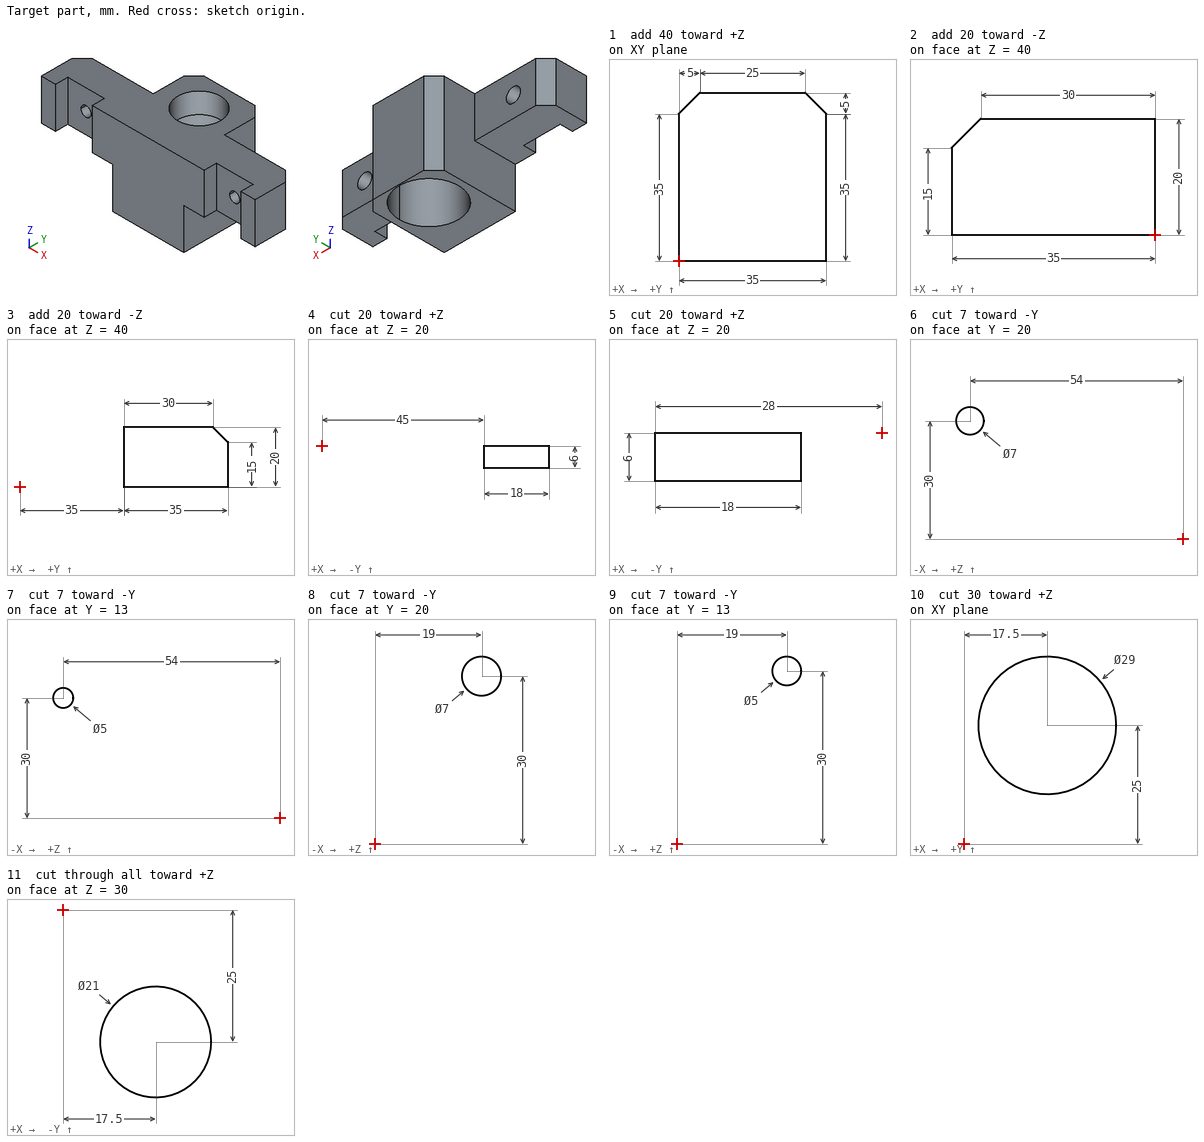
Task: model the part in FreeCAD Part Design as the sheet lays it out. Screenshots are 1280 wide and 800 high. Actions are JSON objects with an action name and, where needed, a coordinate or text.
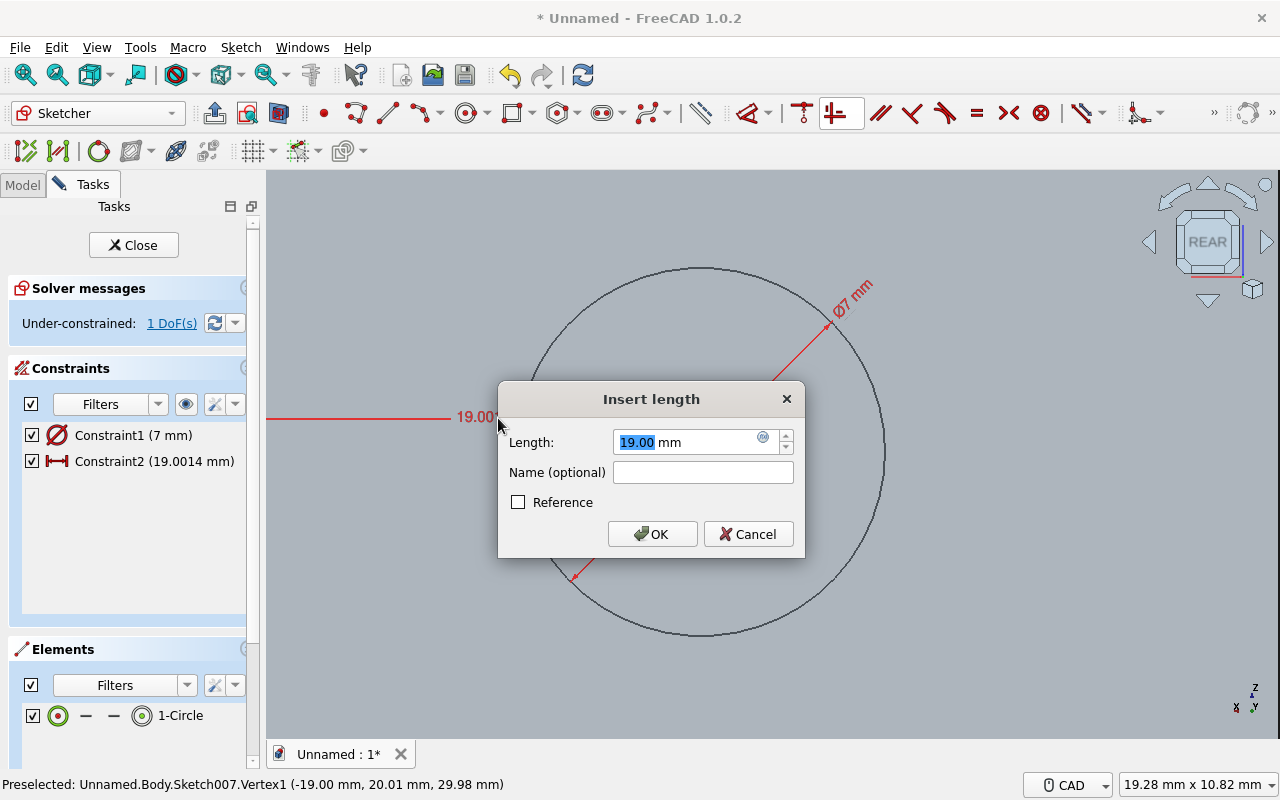
{"action": "type", "text": "19"}
{"action": "key", "text": "Return"}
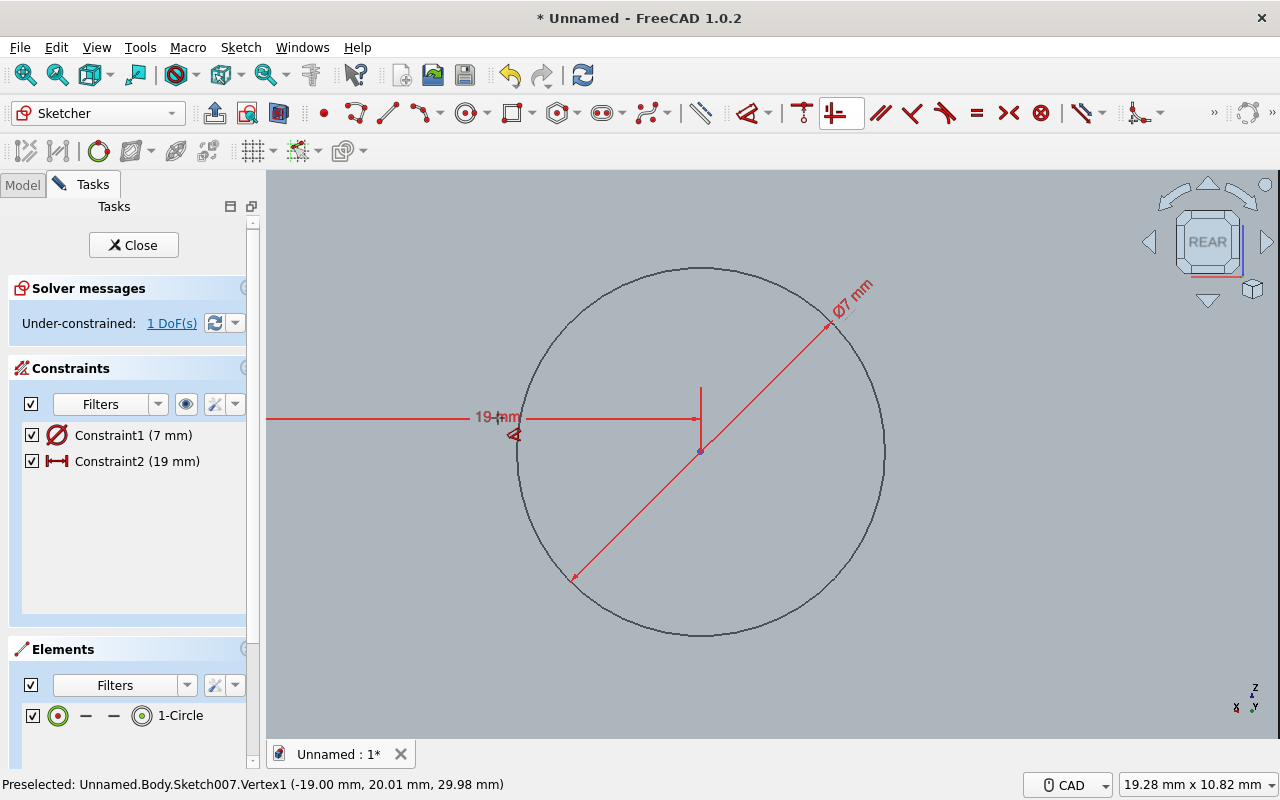
{"action": "left_click", "coordinate": [701, 452]}
{"action": "left_click", "coordinate": [735, 581]}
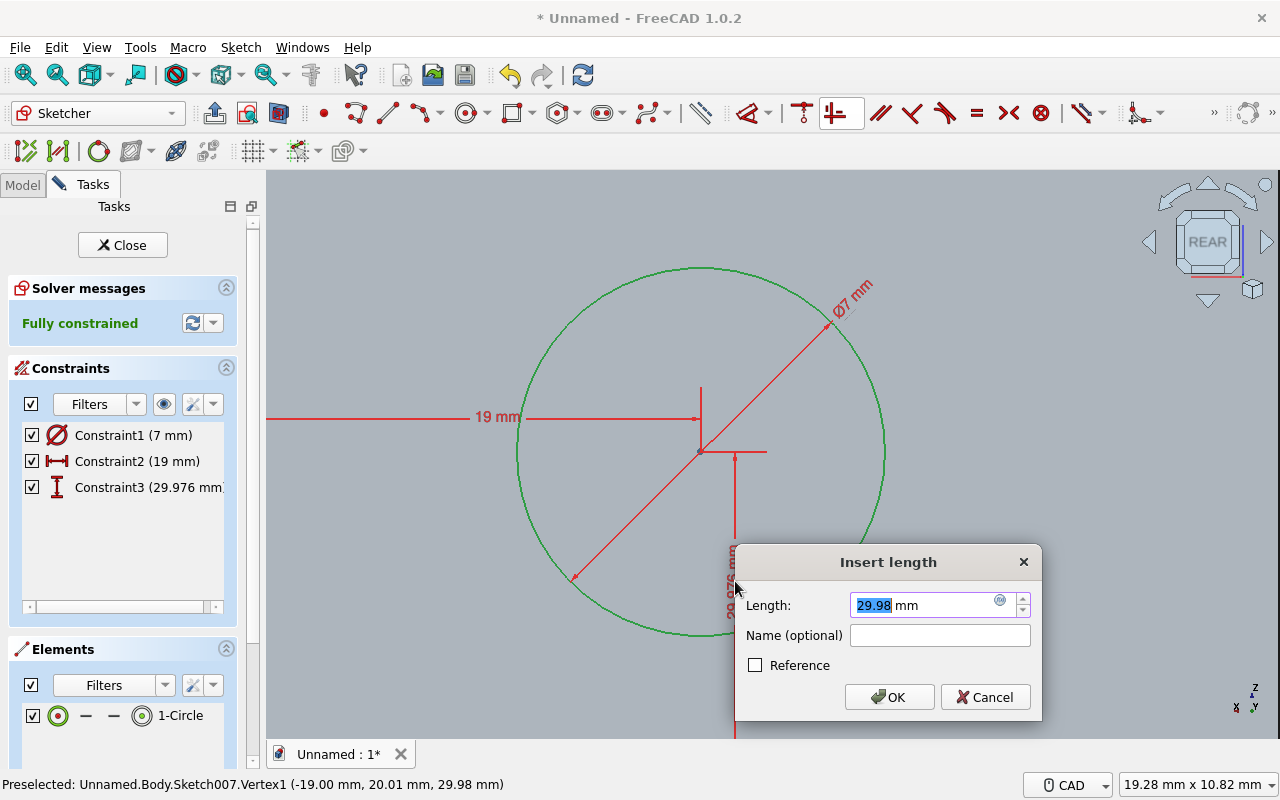
{"action": "type", "text": "30"}
{"action": "key", "text": "Return"}
{"action": "key", "text": "Escape"}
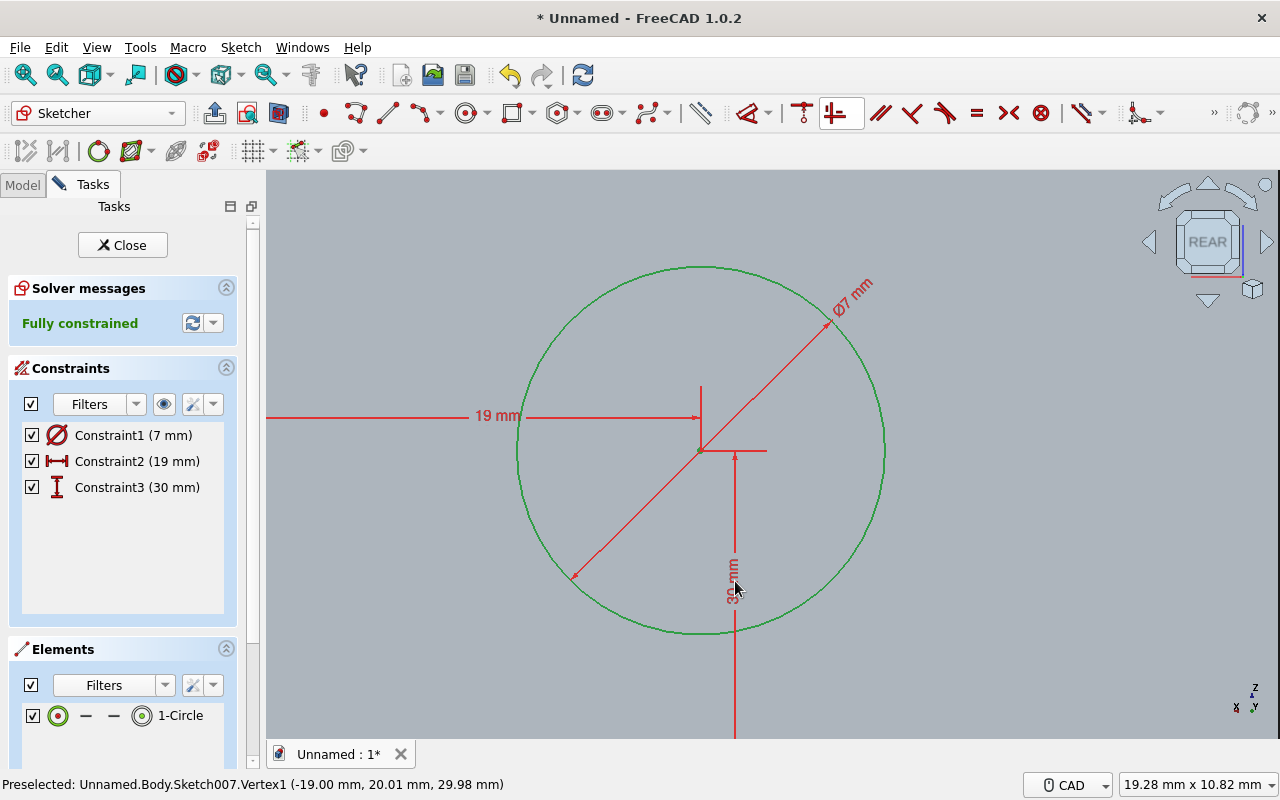
{"action": "left_click", "coordinate": [123, 245]}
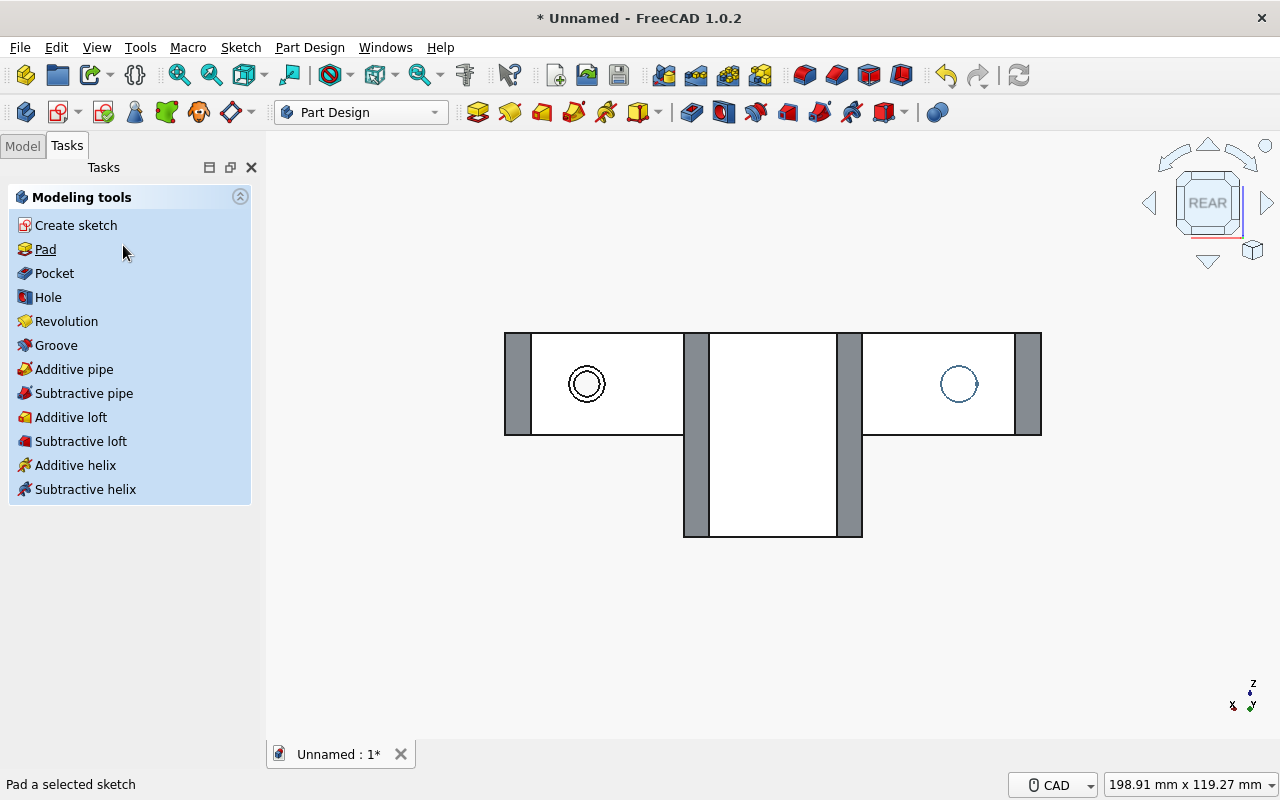
{"action": "left_click", "coordinate": [692, 112]}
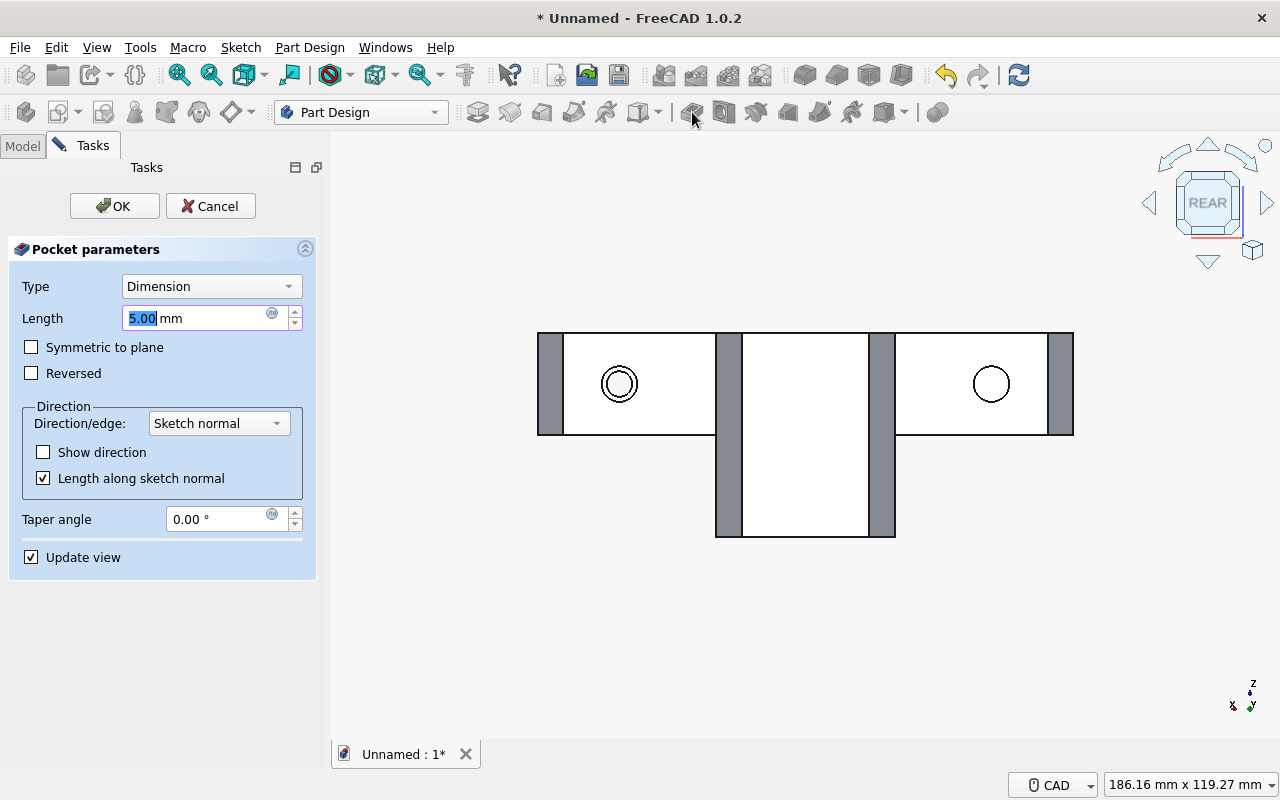
{"action": "type", "text": "7"}
{"action": "key", "text": "Tab"}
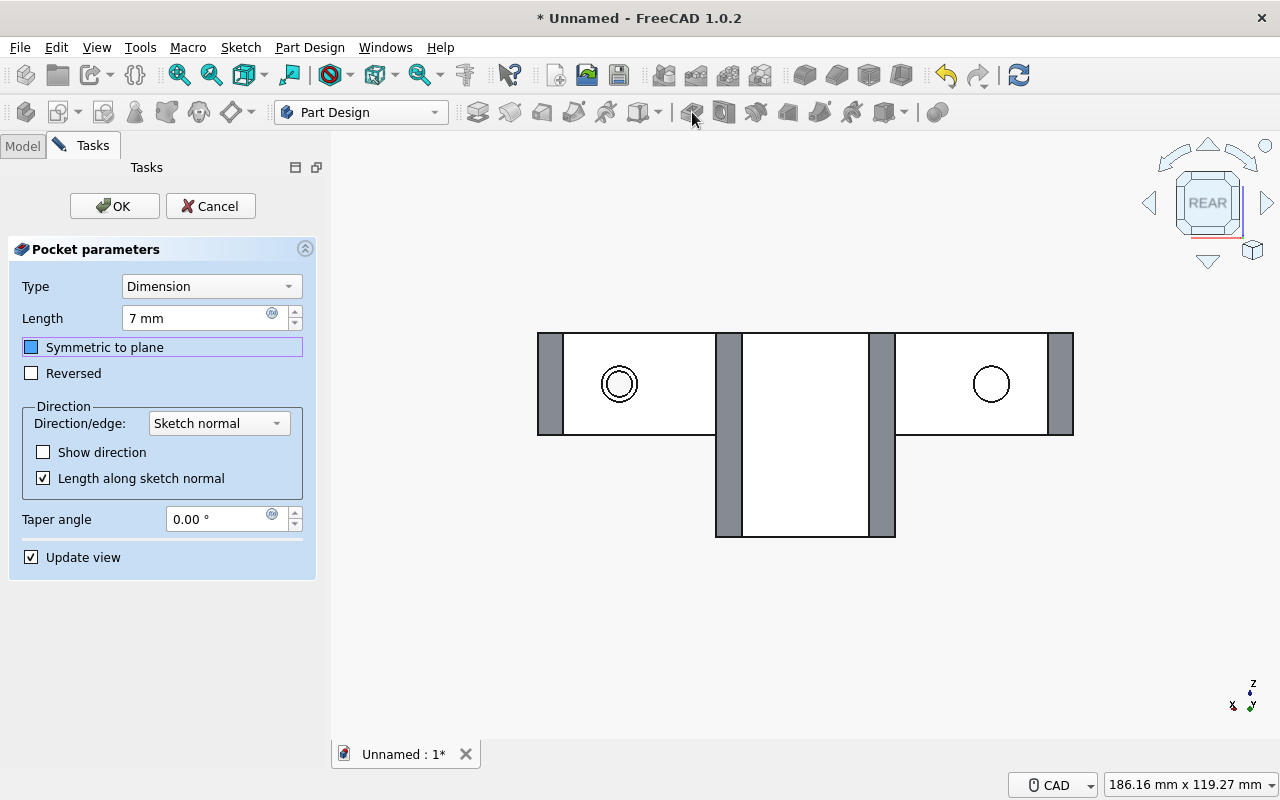
{"action": "left_click", "coordinate": [115, 206]}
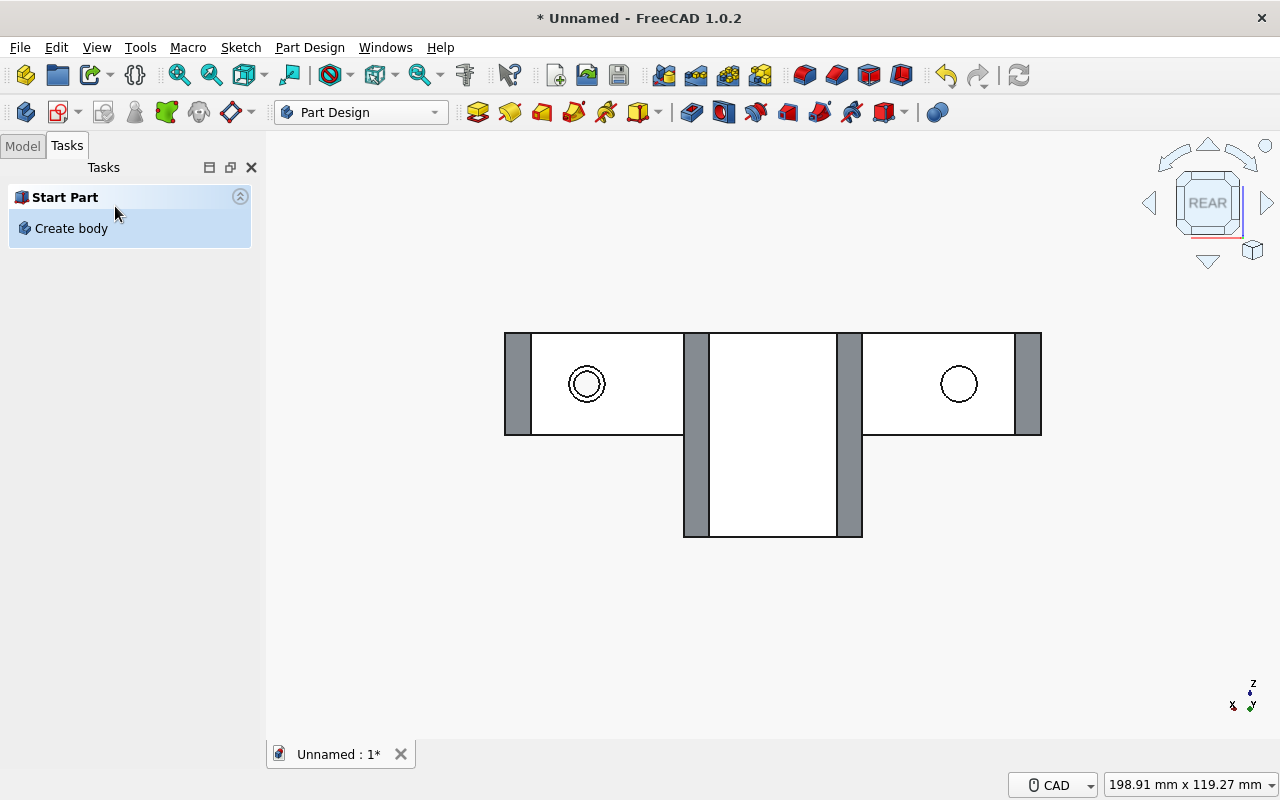
{"action": "left_click", "coordinate": [959, 383]}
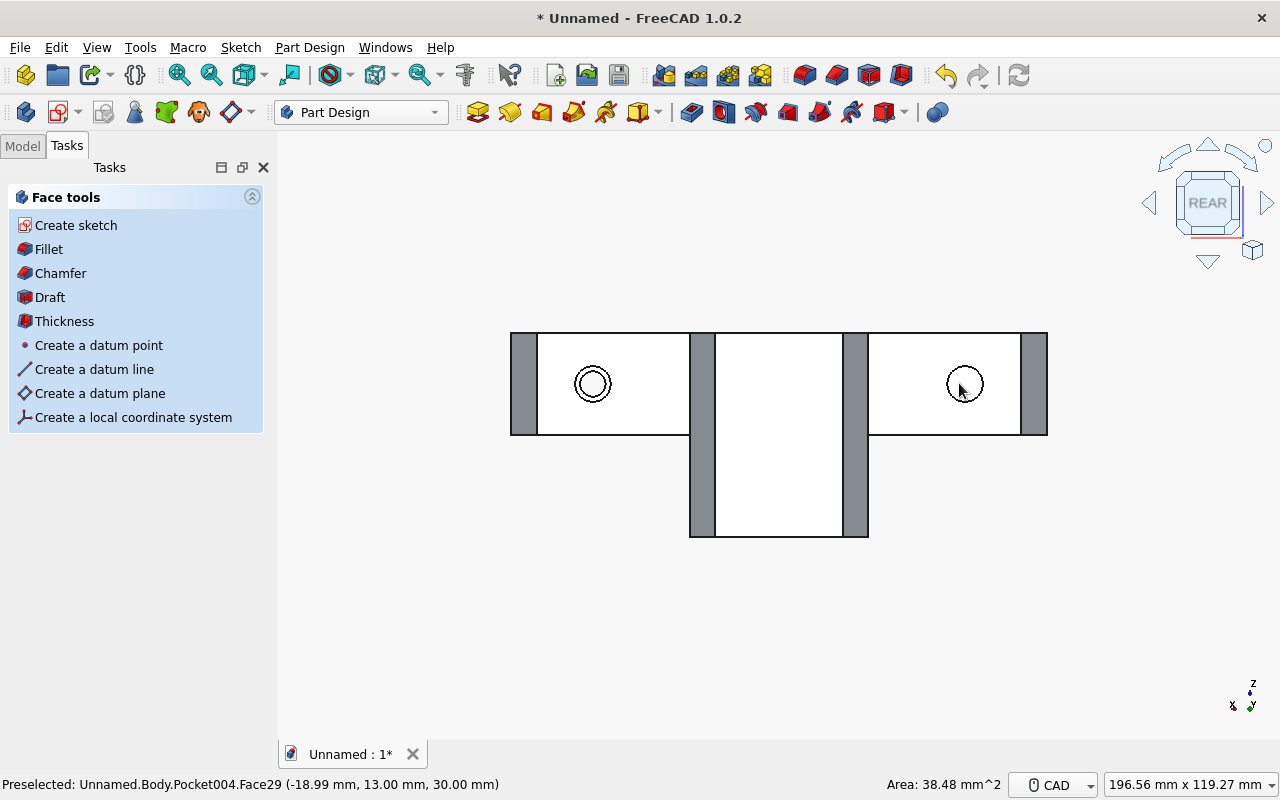
{"action": "left_click", "coordinate": [58, 112]}